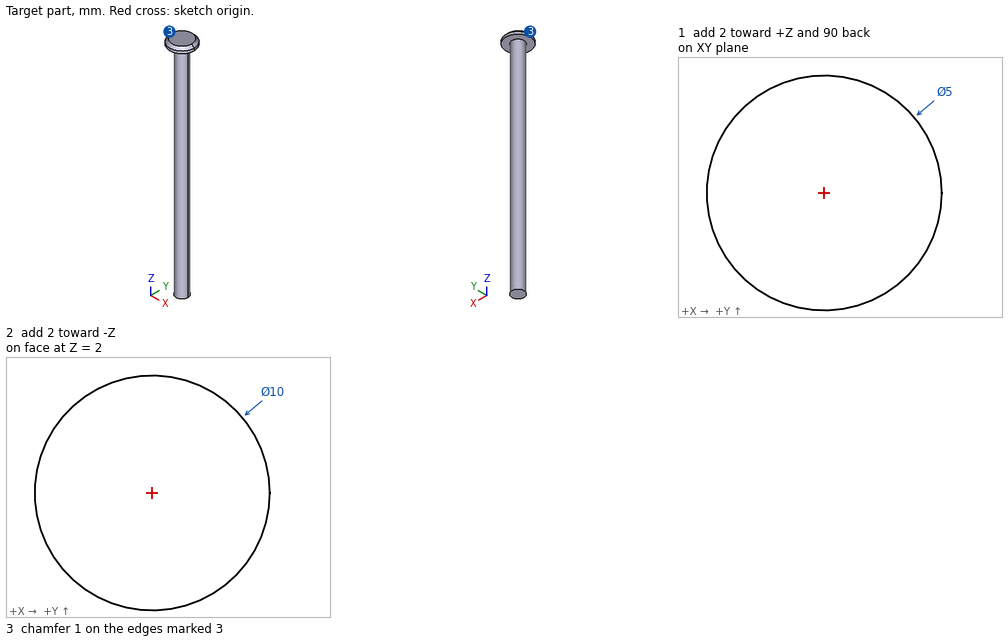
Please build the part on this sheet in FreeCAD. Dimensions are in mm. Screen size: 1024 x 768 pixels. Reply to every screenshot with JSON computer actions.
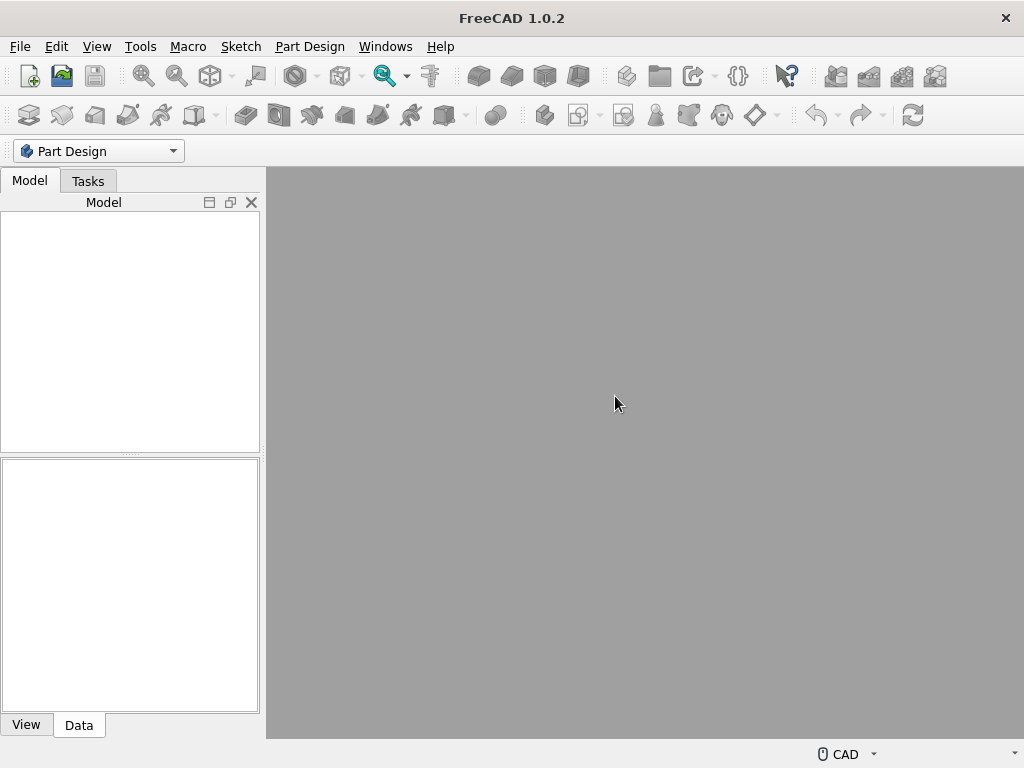
{"action": "key", "text": "ctrl+n"}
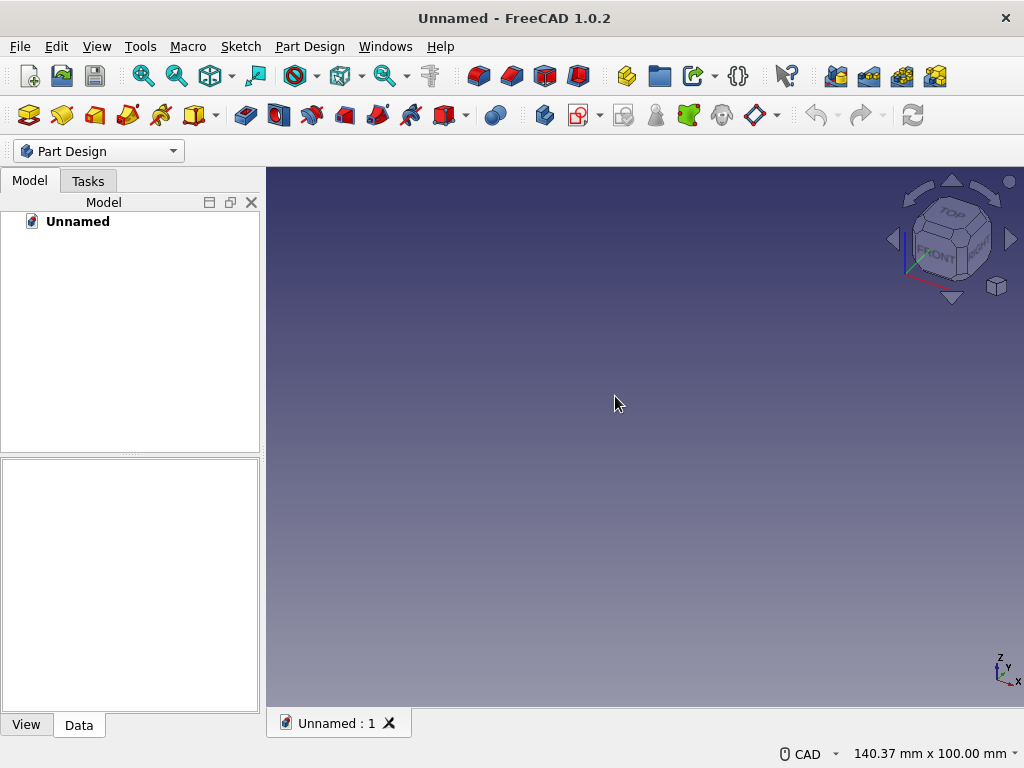
{"action": "left_click", "coordinate": [578, 116]}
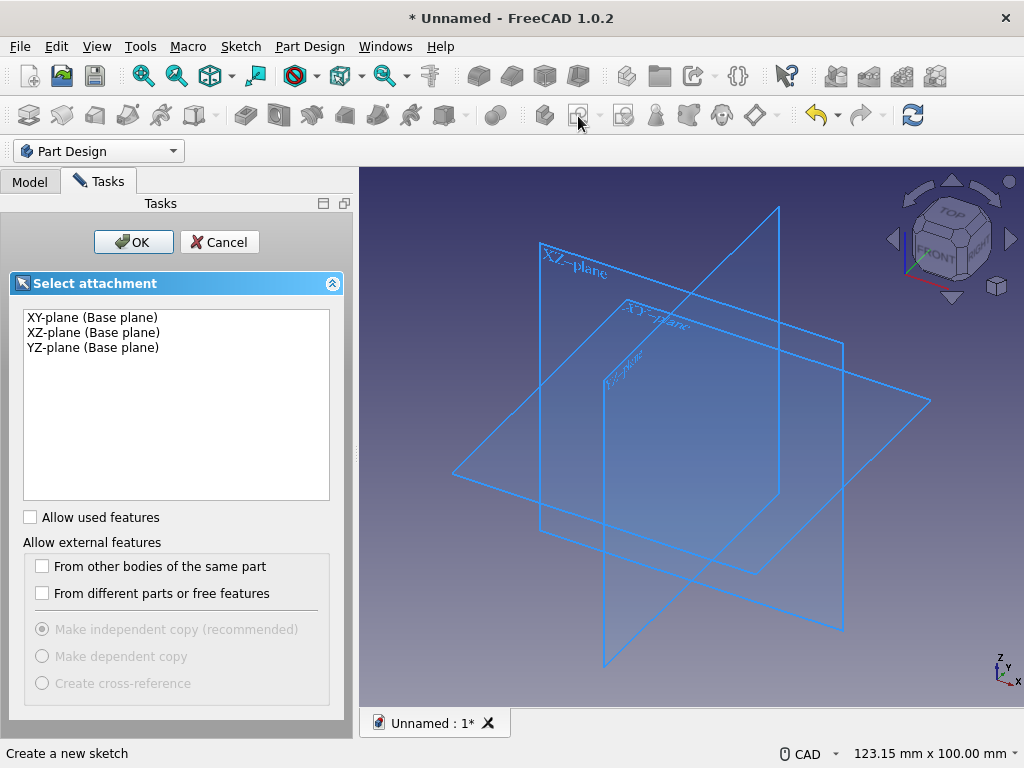
{"action": "left_click", "coordinate": [84, 318]}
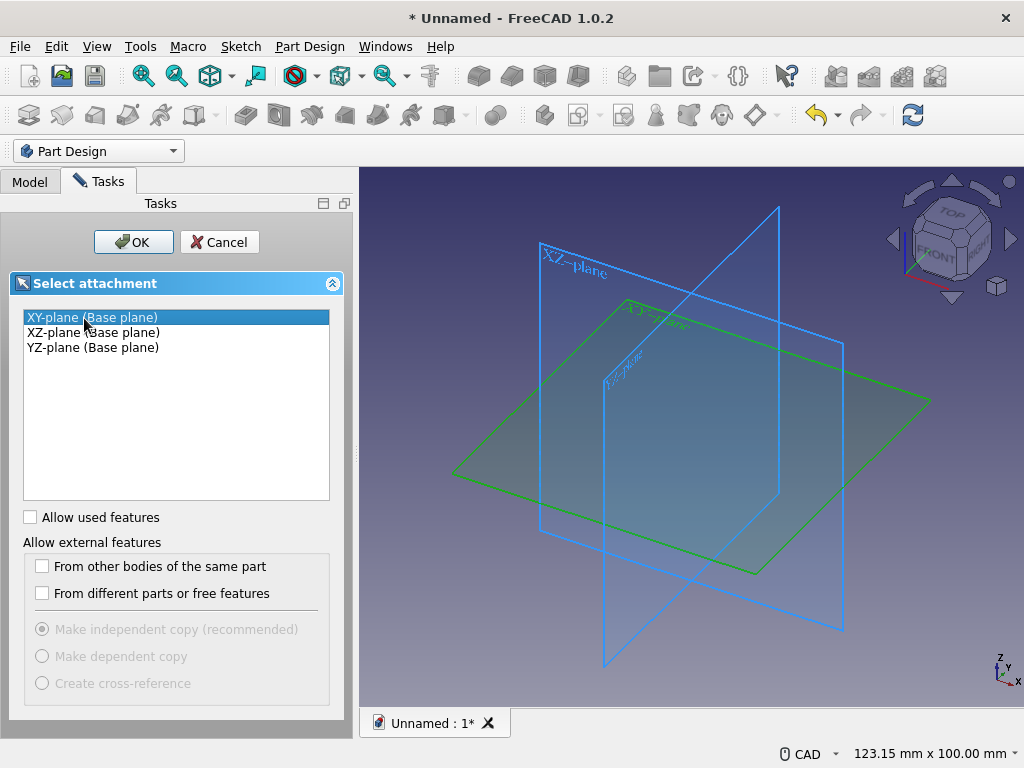
{"action": "left_click", "coordinate": [134, 242]}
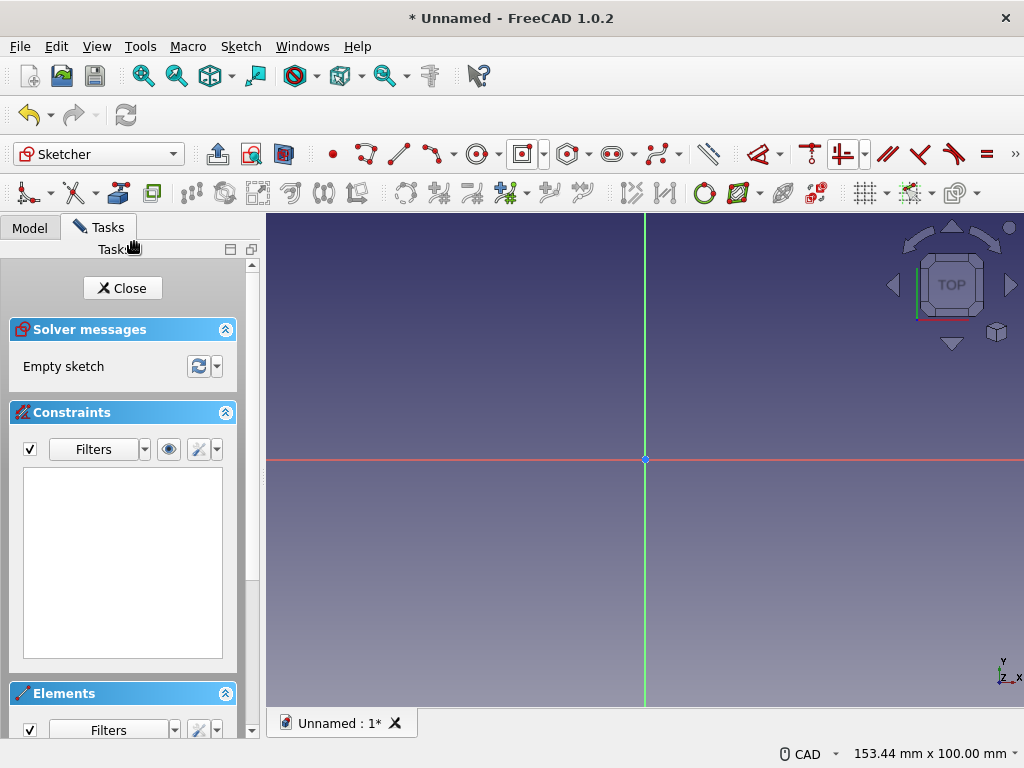
{"action": "scroll", "coordinate": [650, 460], "scroll_direction": "up", "scroll_amount": 13}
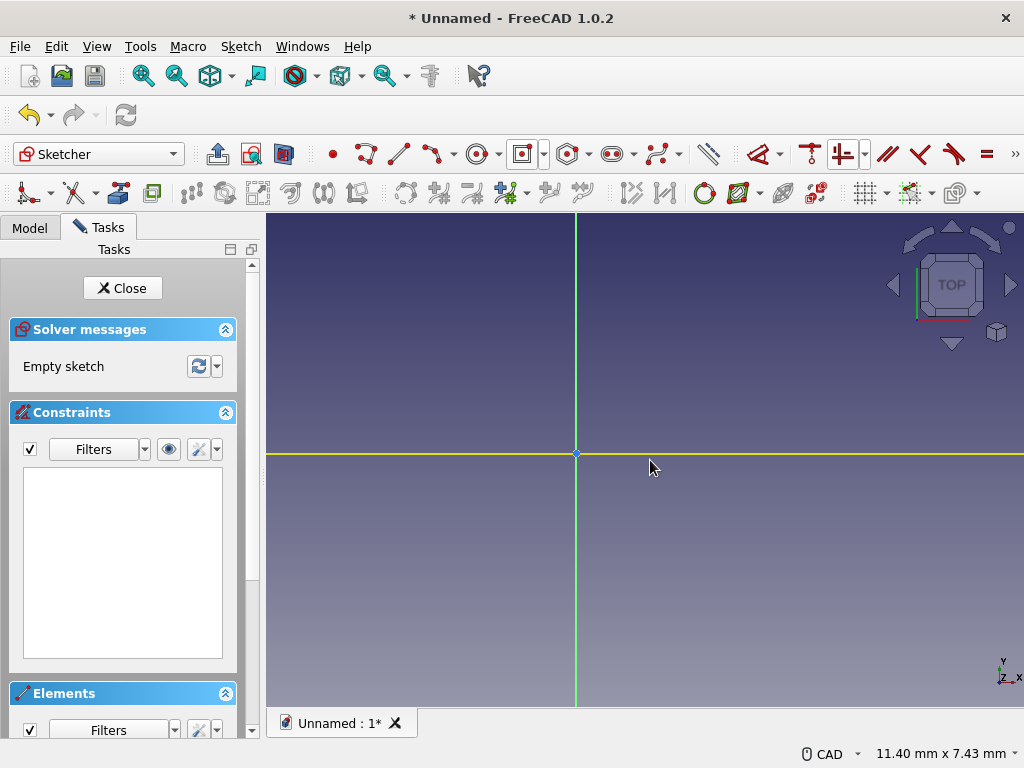
{"action": "left_click", "coordinate": [476, 154]}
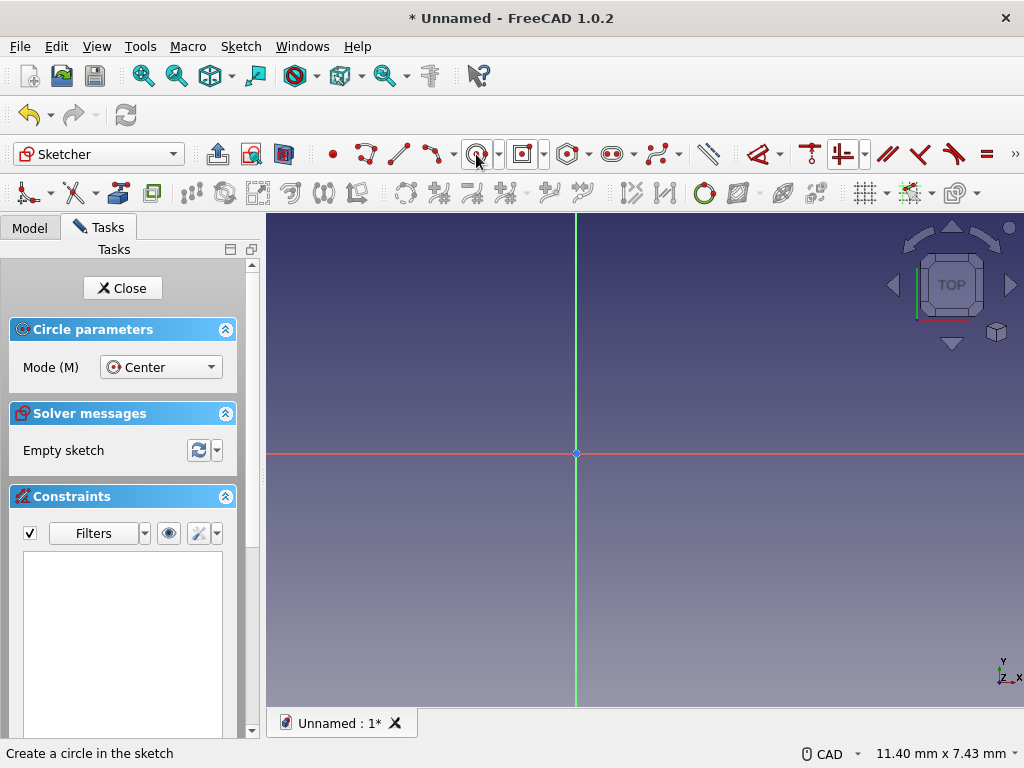
{"action": "left_click", "coordinate": [576, 454]}
{"action": "mouse_move", "coordinate": [694, 336]}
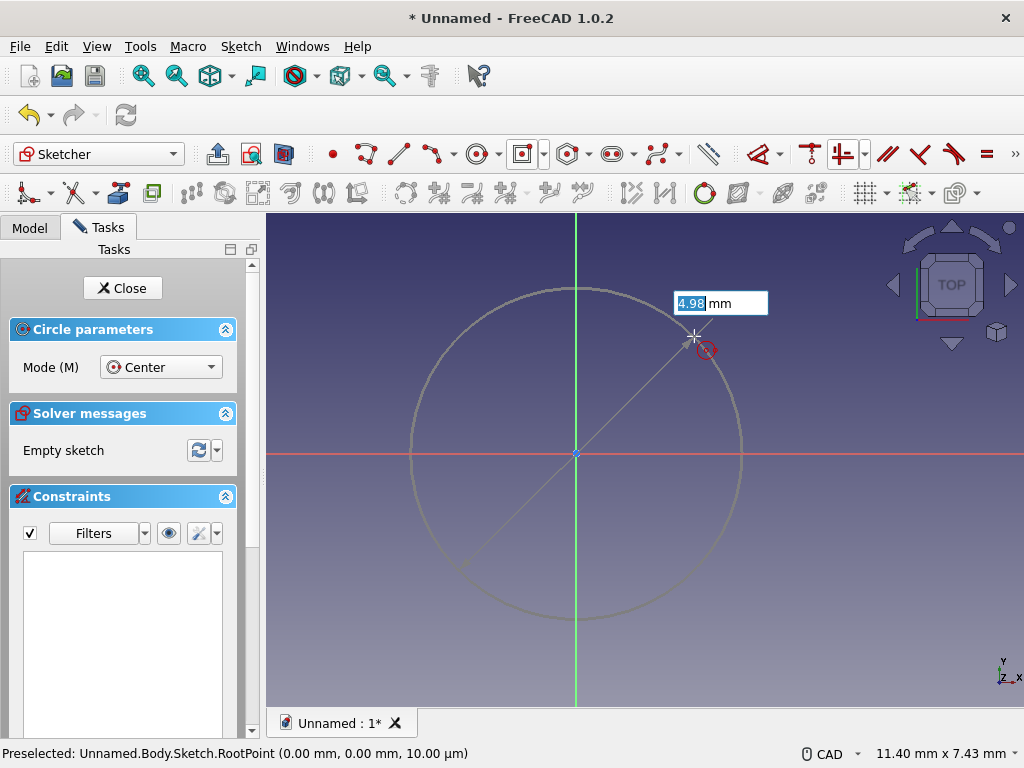
{"action": "type", "text": "5"}
{"action": "key", "text": "Return"}
{"action": "key", "text": "Escape"}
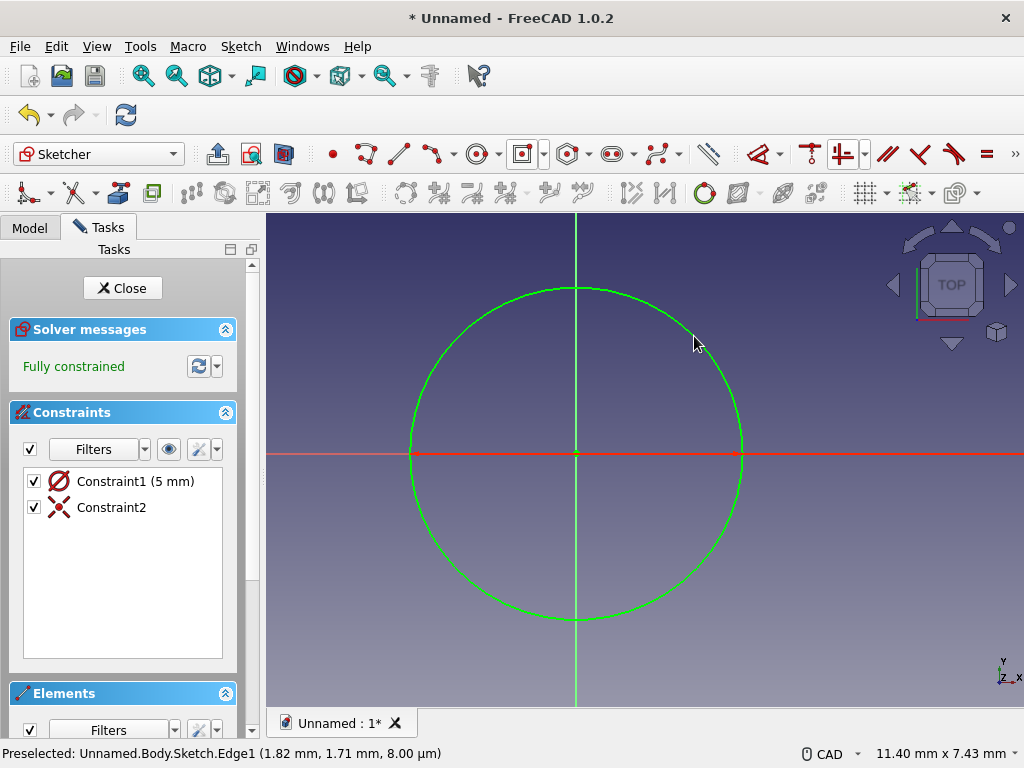
{"action": "left_click", "coordinate": [123, 288]}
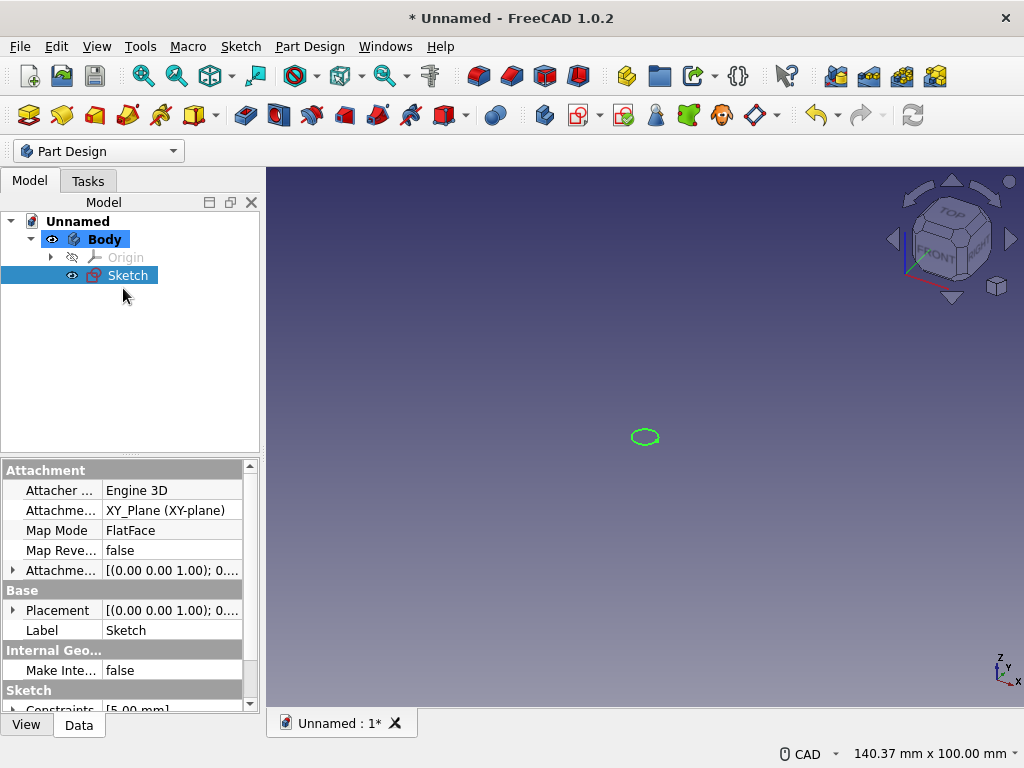
{"action": "left_click", "coordinate": [29, 116]}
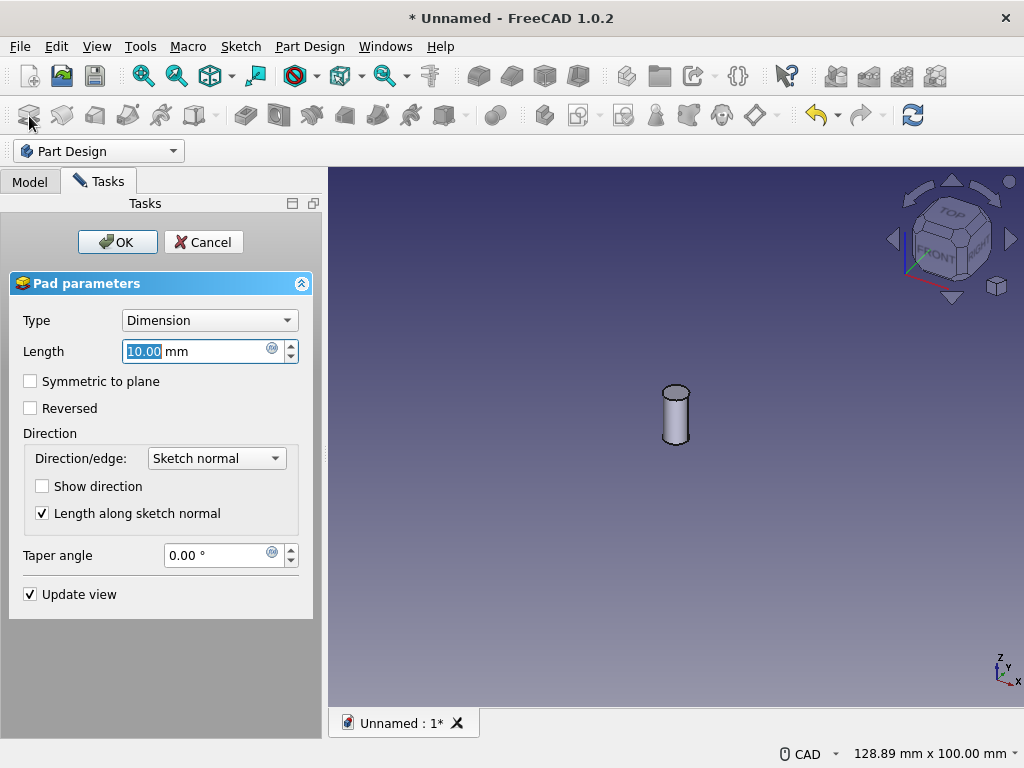
{"action": "left_click", "coordinate": [210, 320]}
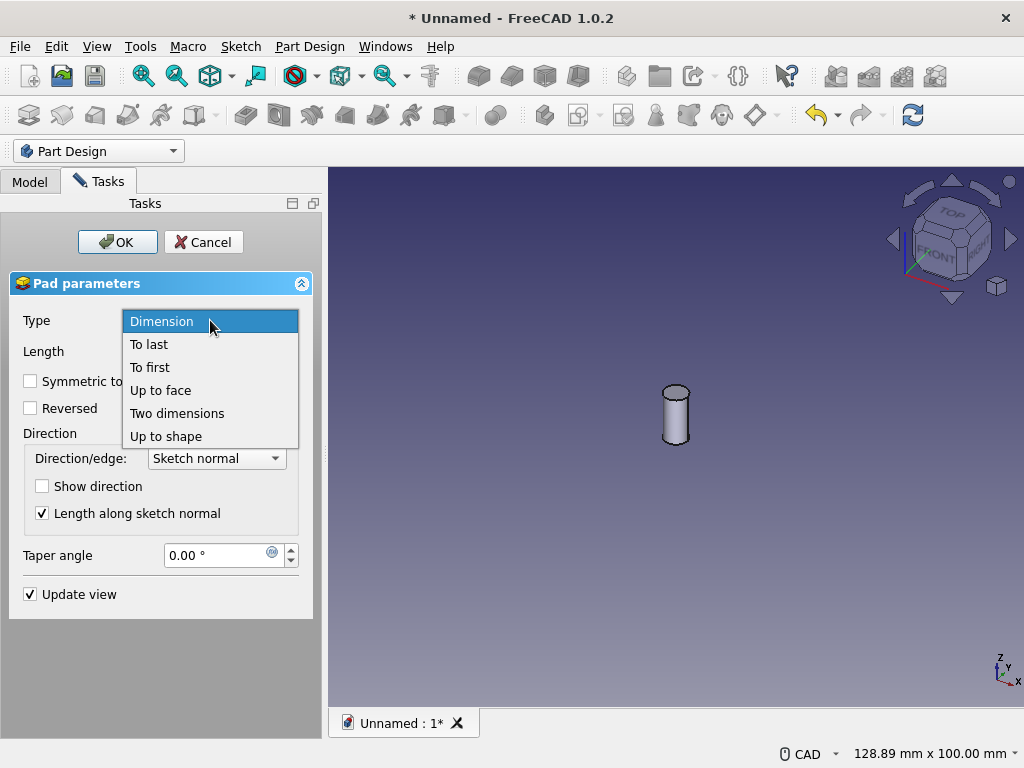
{"action": "left_click", "coordinate": [208, 414]}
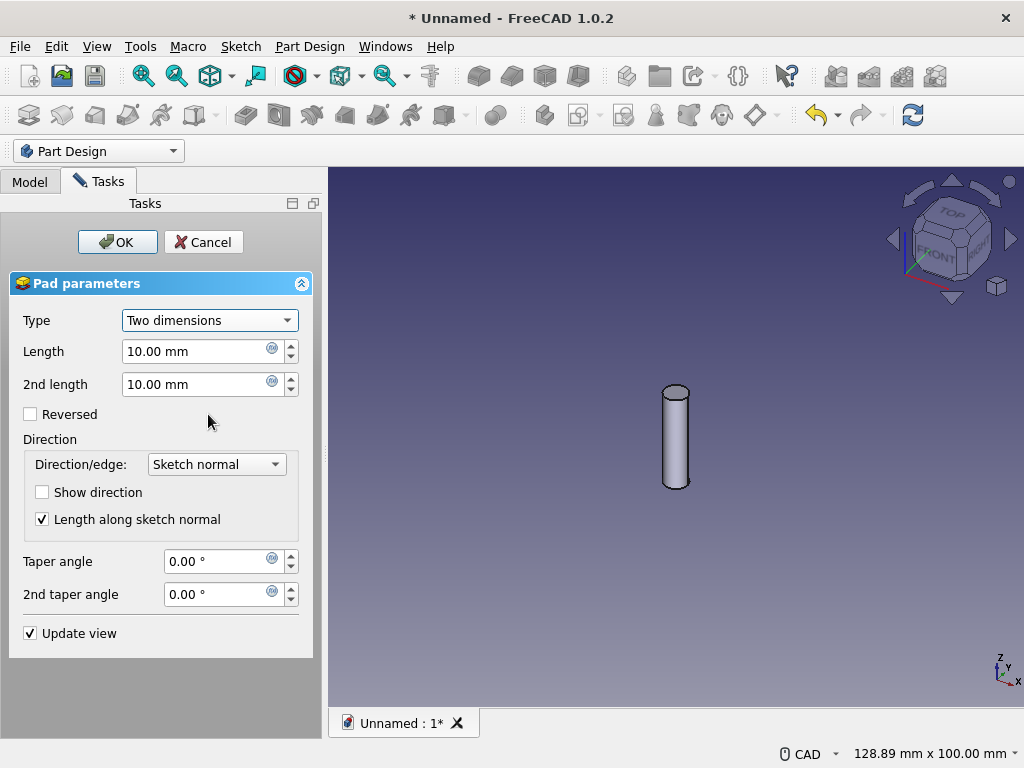
{"action": "triple_click", "coordinate": [204, 352]}